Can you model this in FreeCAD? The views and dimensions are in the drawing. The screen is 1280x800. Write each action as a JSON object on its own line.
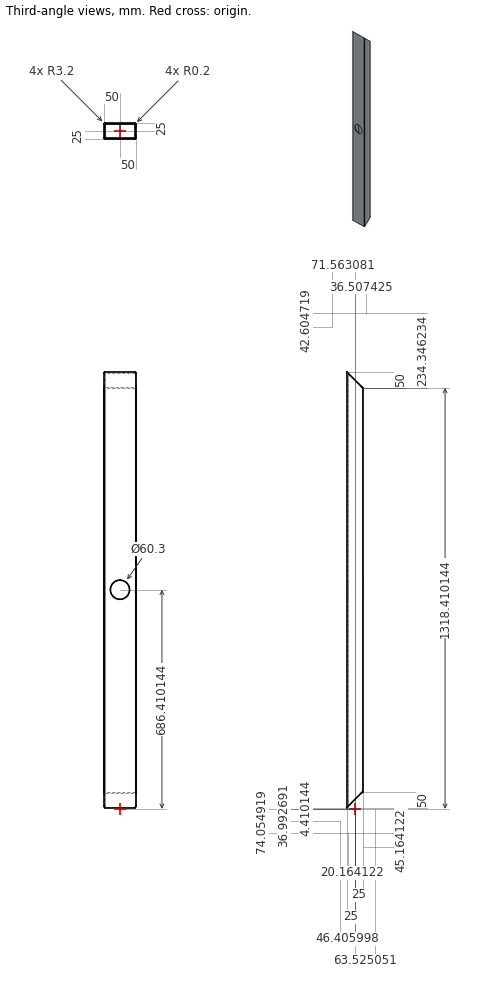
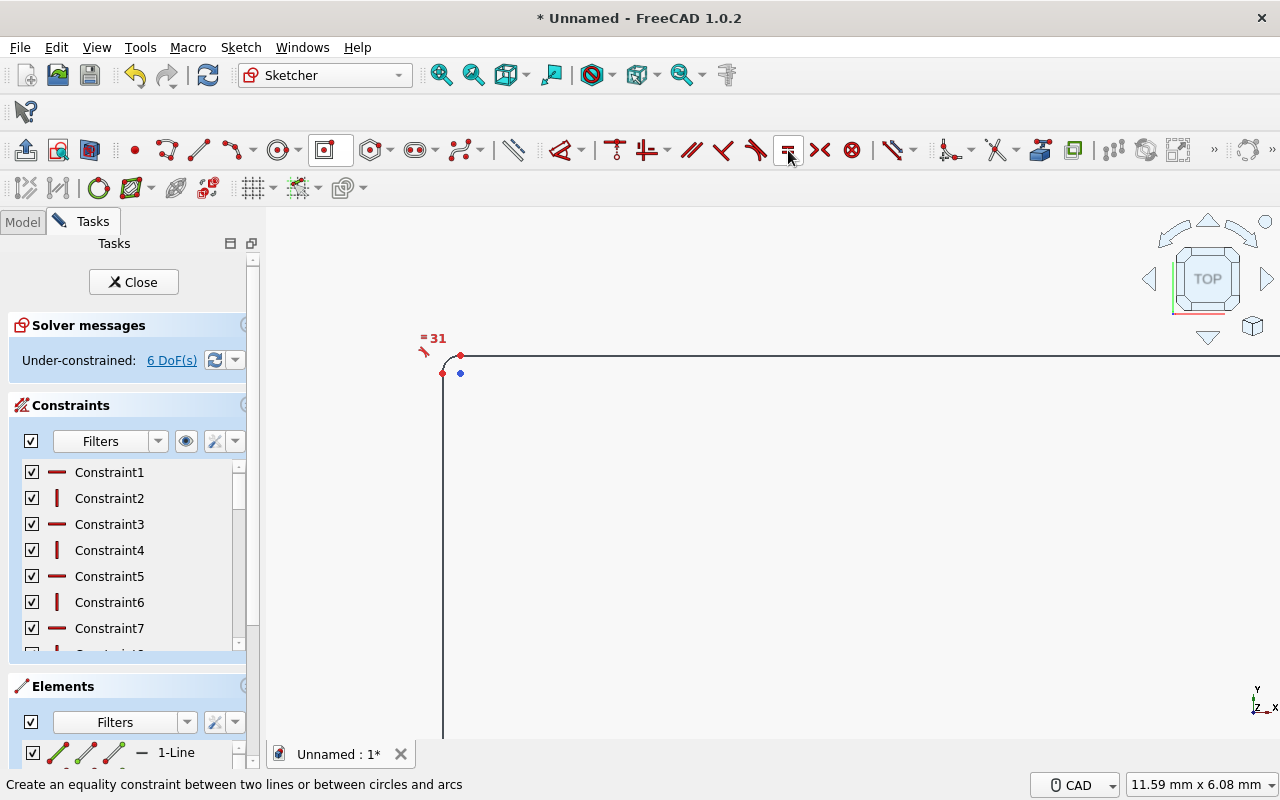
{"action": "left_click", "coordinate": [560, 150]}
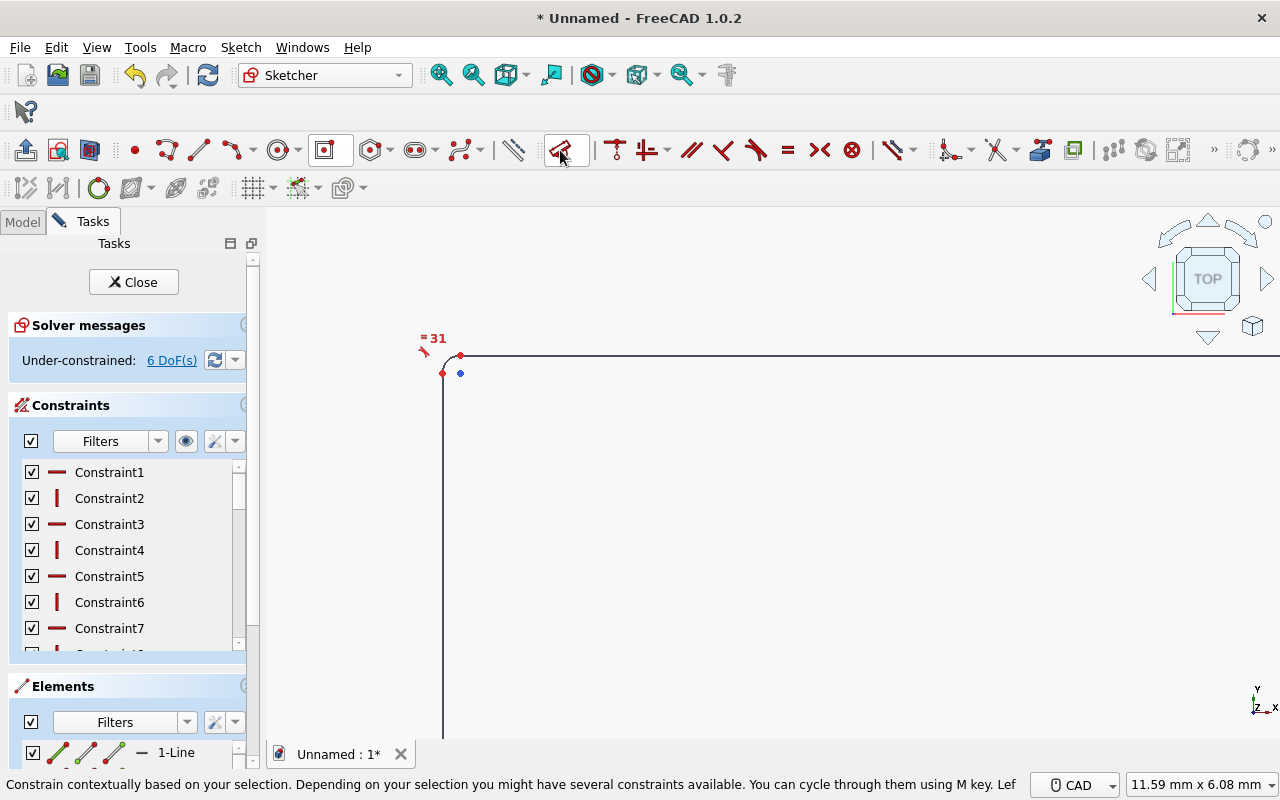
{"action": "scroll", "coordinate": [455, 357], "scroll_direction": "down", "scroll_amount": 14}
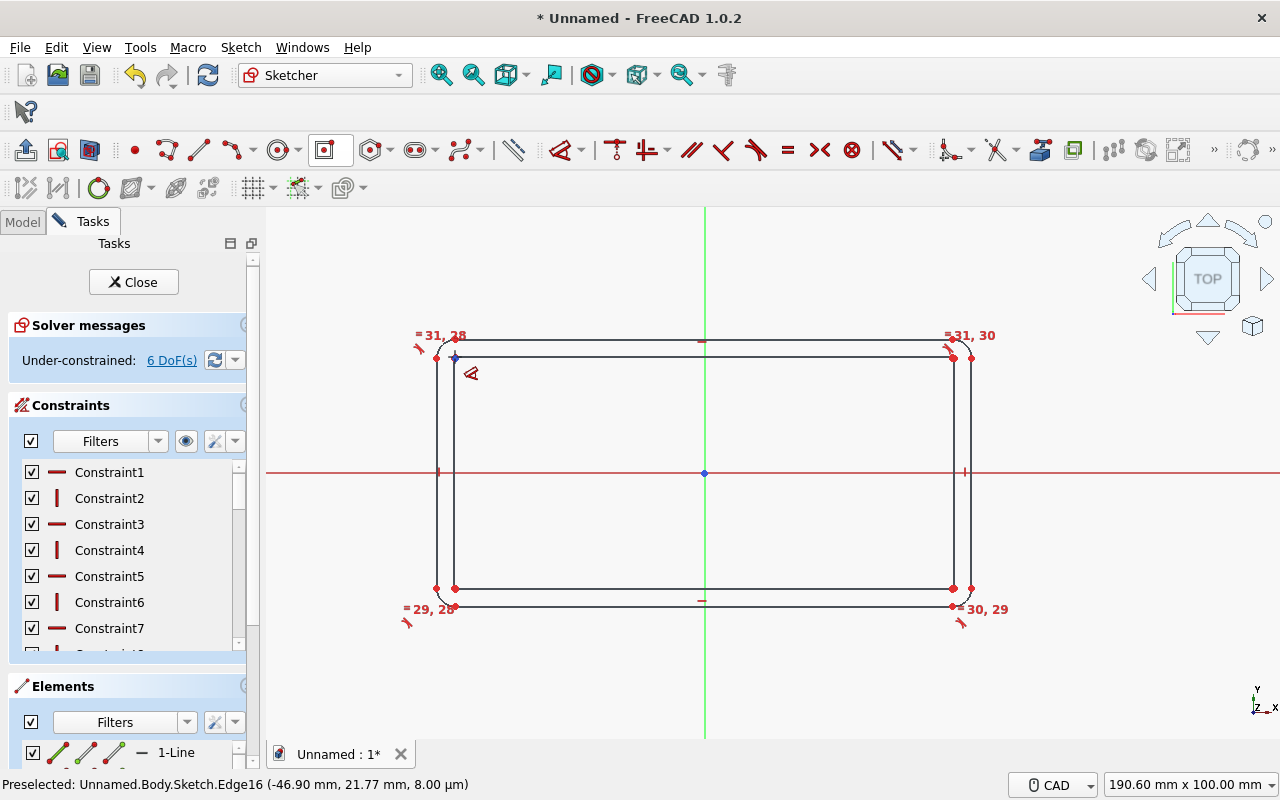
{"action": "scroll", "coordinate": [447, 342], "scroll_direction": "up", "scroll_amount": 5}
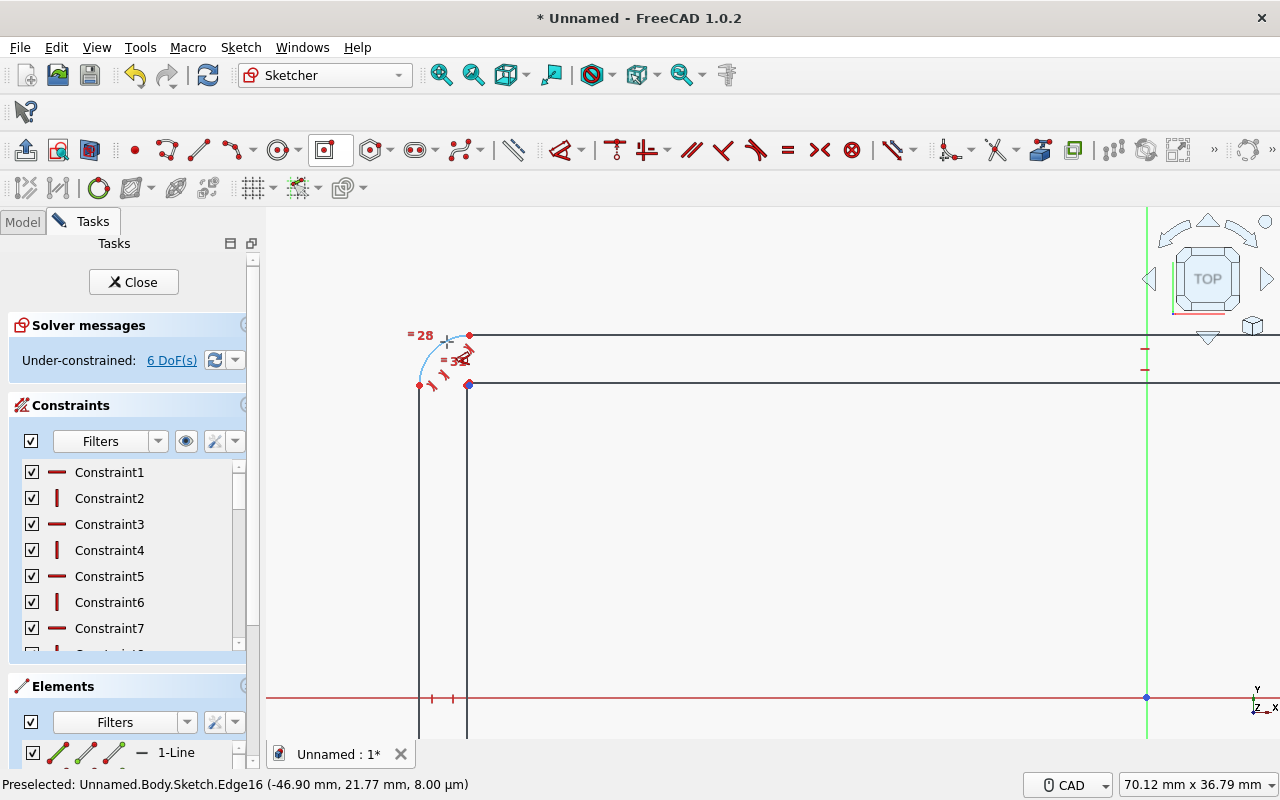
{"action": "left_click", "coordinate": [447, 341]}
{"action": "left_click", "coordinate": [432, 312]}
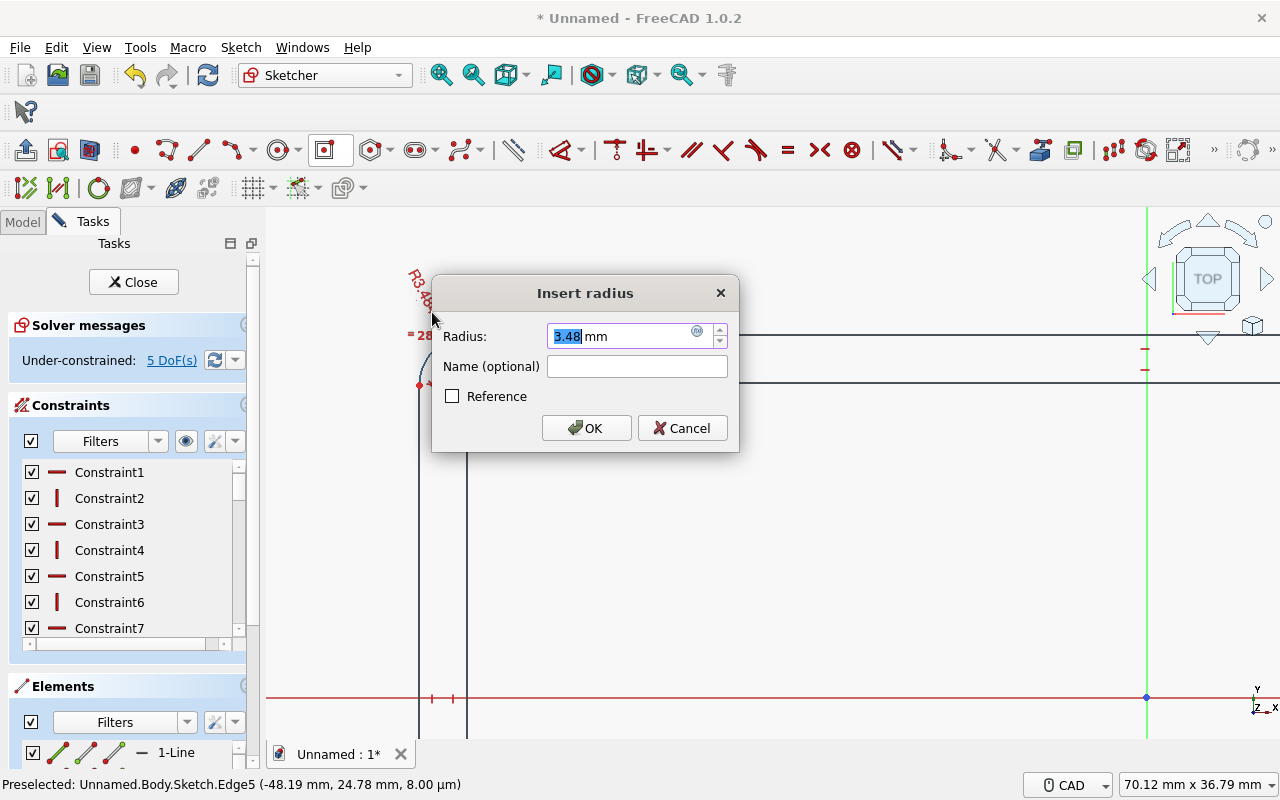
{"action": "type", "text": "3.2"}
{"action": "key", "text": "Return"}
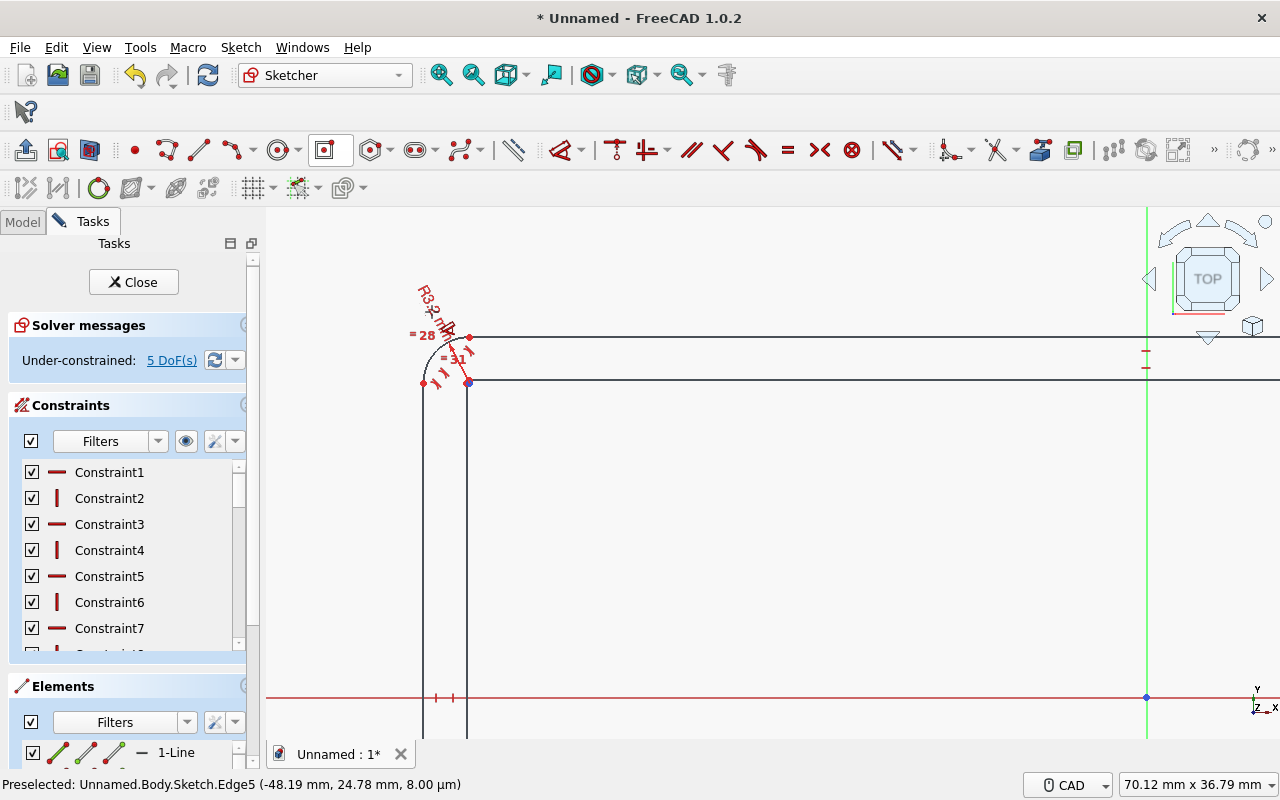
{"action": "scroll", "coordinate": [447, 342], "scroll_direction": "down", "scroll_amount": 5}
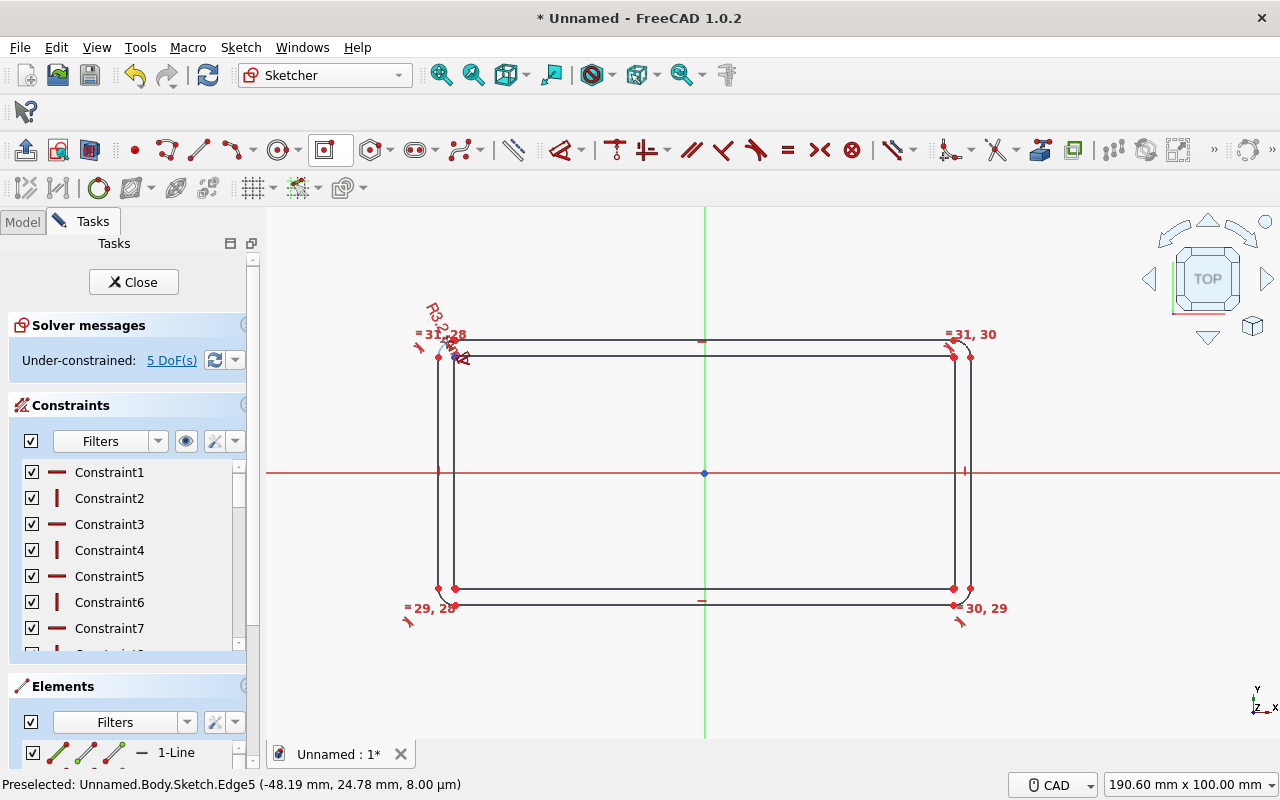
{"action": "scroll", "coordinate": [954, 357], "scroll_direction": "up", "scroll_amount": 19}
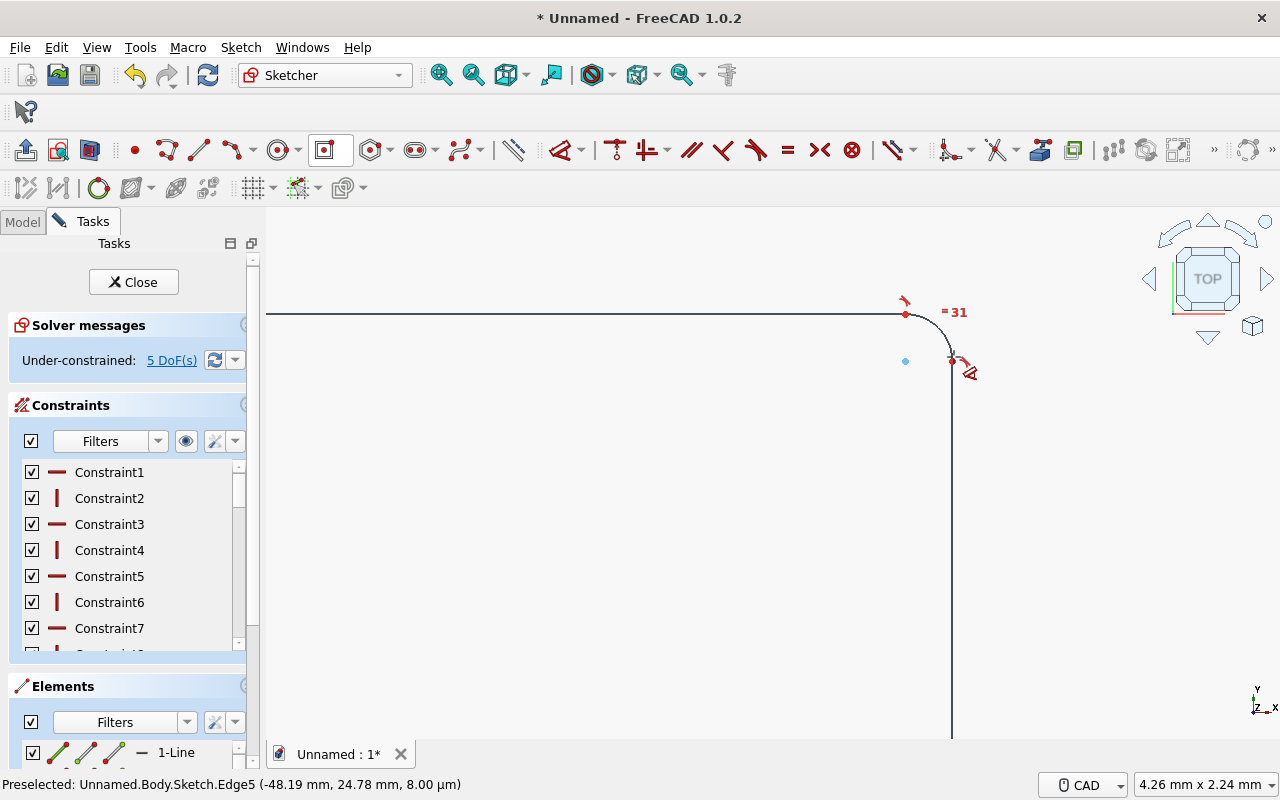
{"action": "left_click", "coordinate": [938, 328]}
{"action": "left_click", "coordinate": [960, 305]}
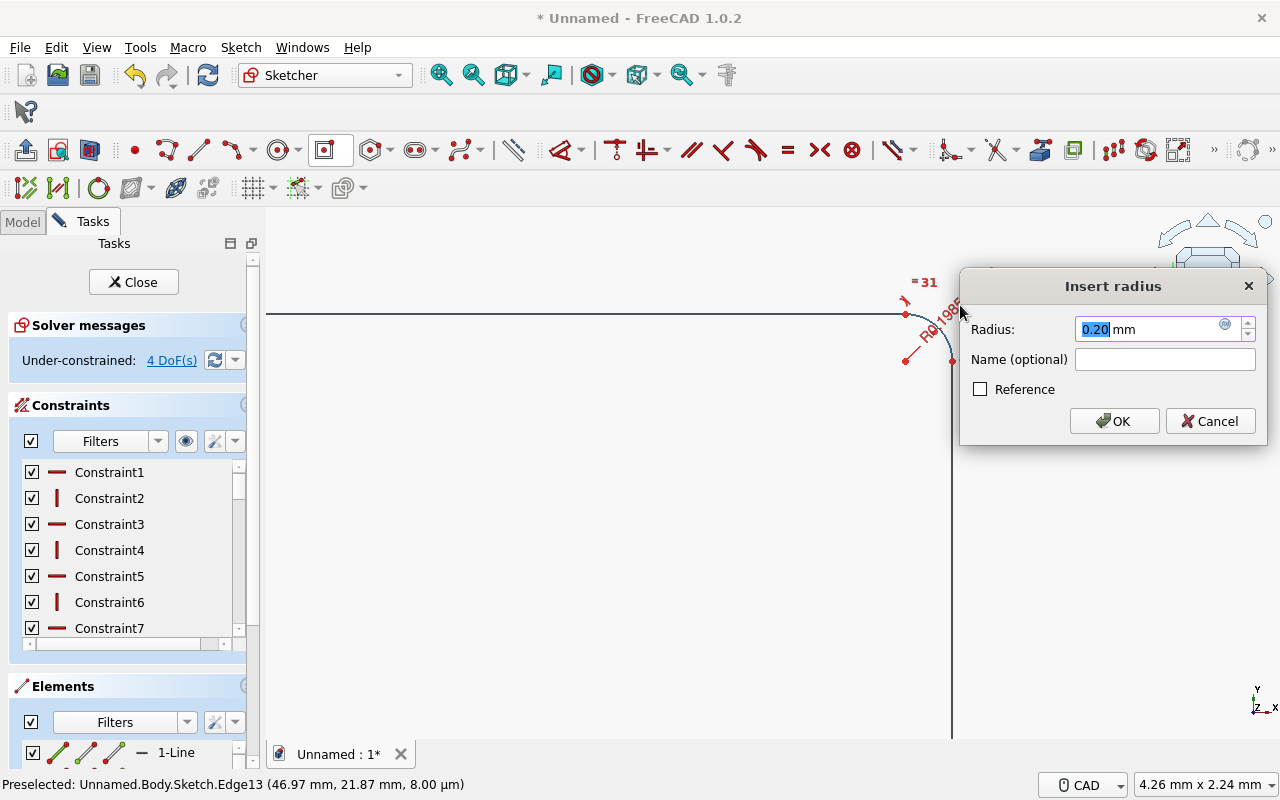
{"action": "type", "text": "0.2"}
{"action": "key", "text": "Return"}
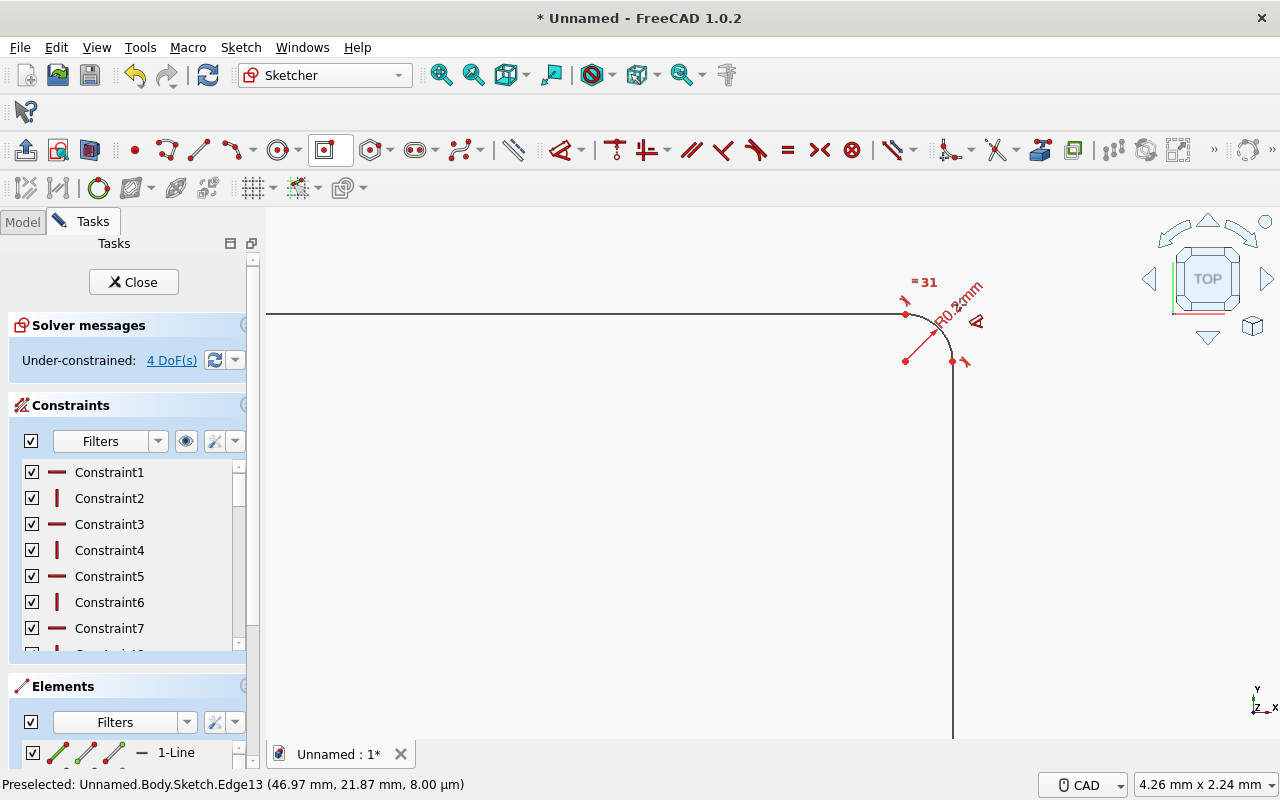
{"action": "scroll", "coordinate": [1012, 331], "scroll_direction": "down", "scroll_amount": 18}